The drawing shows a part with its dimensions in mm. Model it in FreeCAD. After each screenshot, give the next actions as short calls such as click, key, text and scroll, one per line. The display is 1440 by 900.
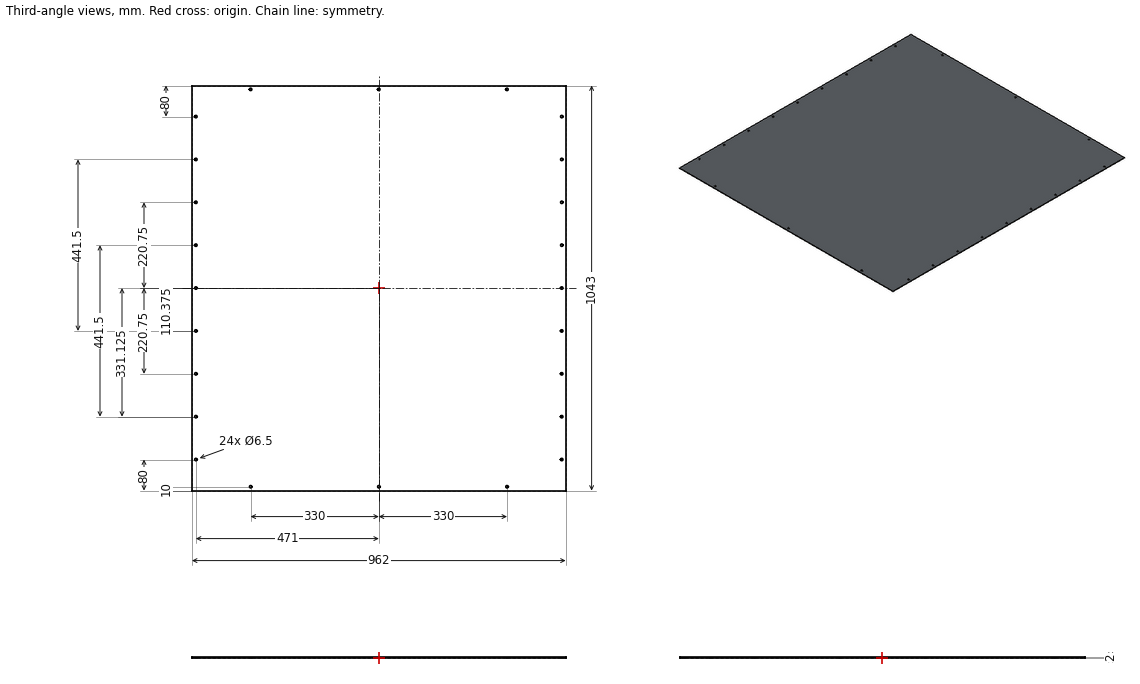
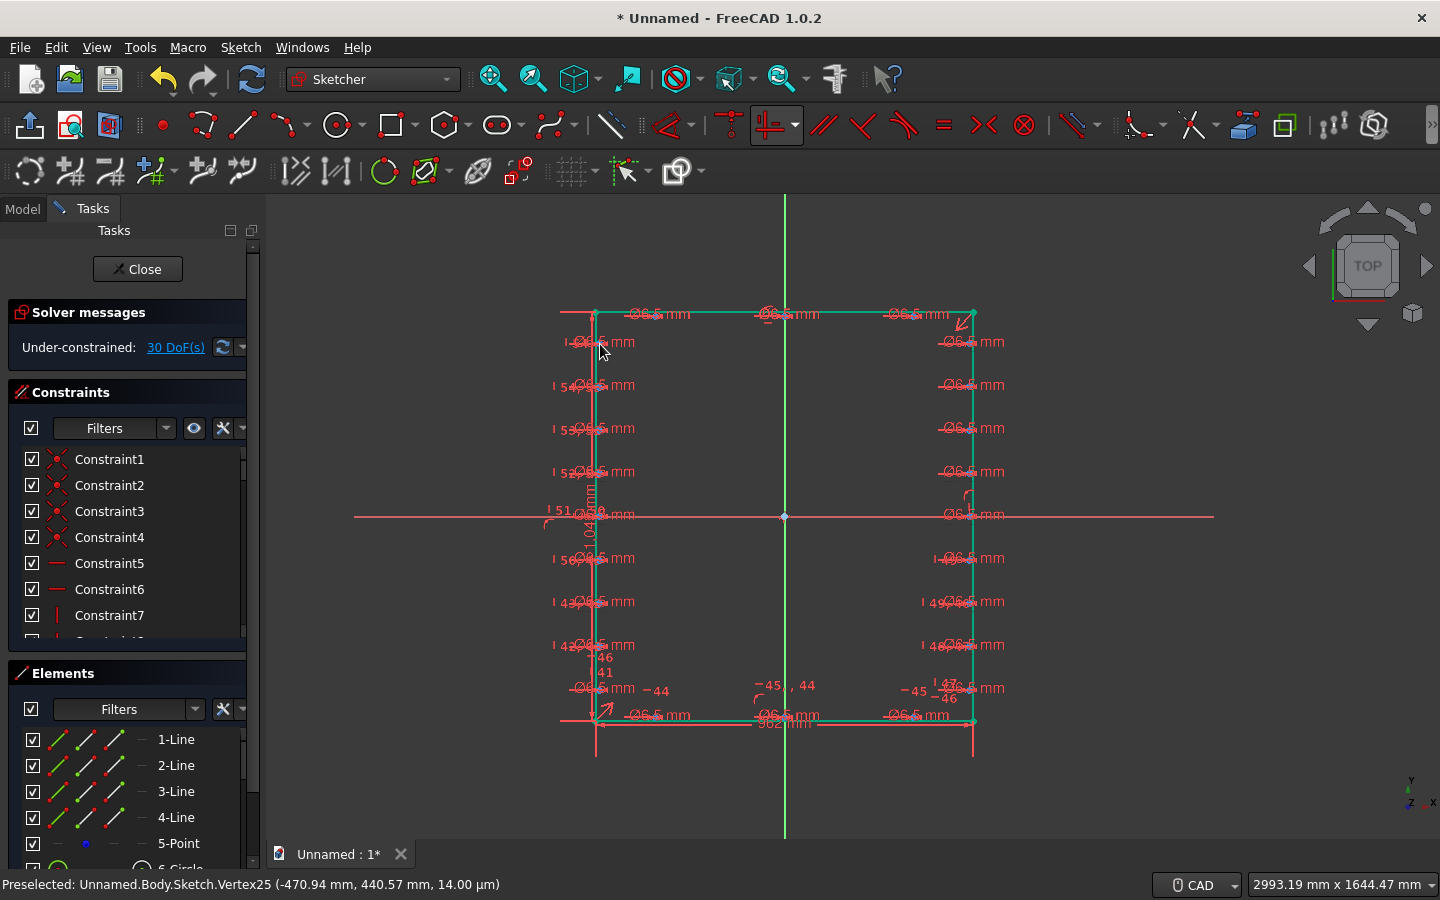
click(969, 560)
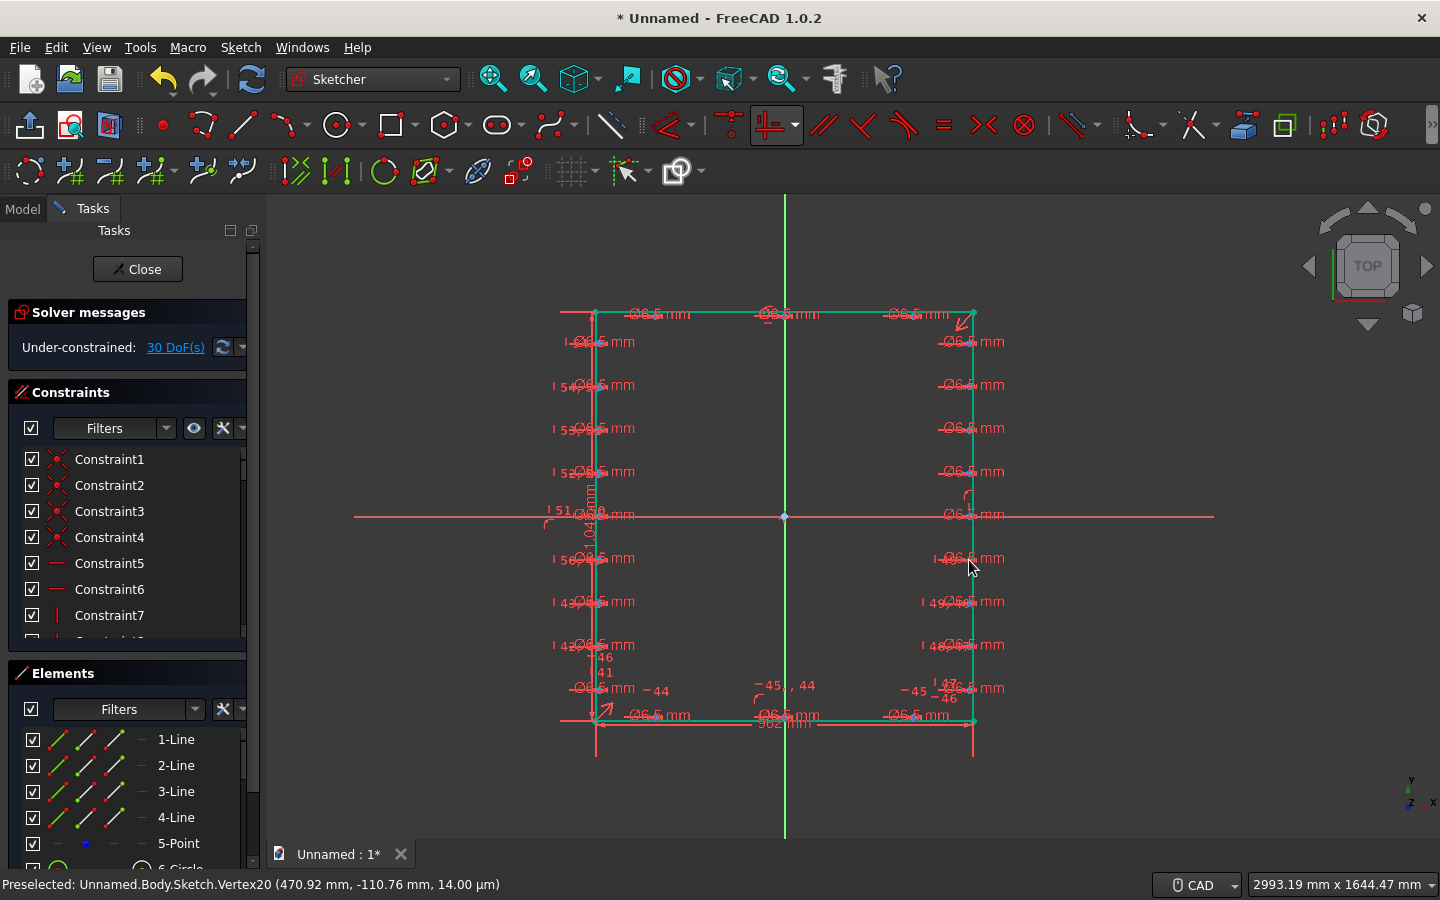
click(969, 517)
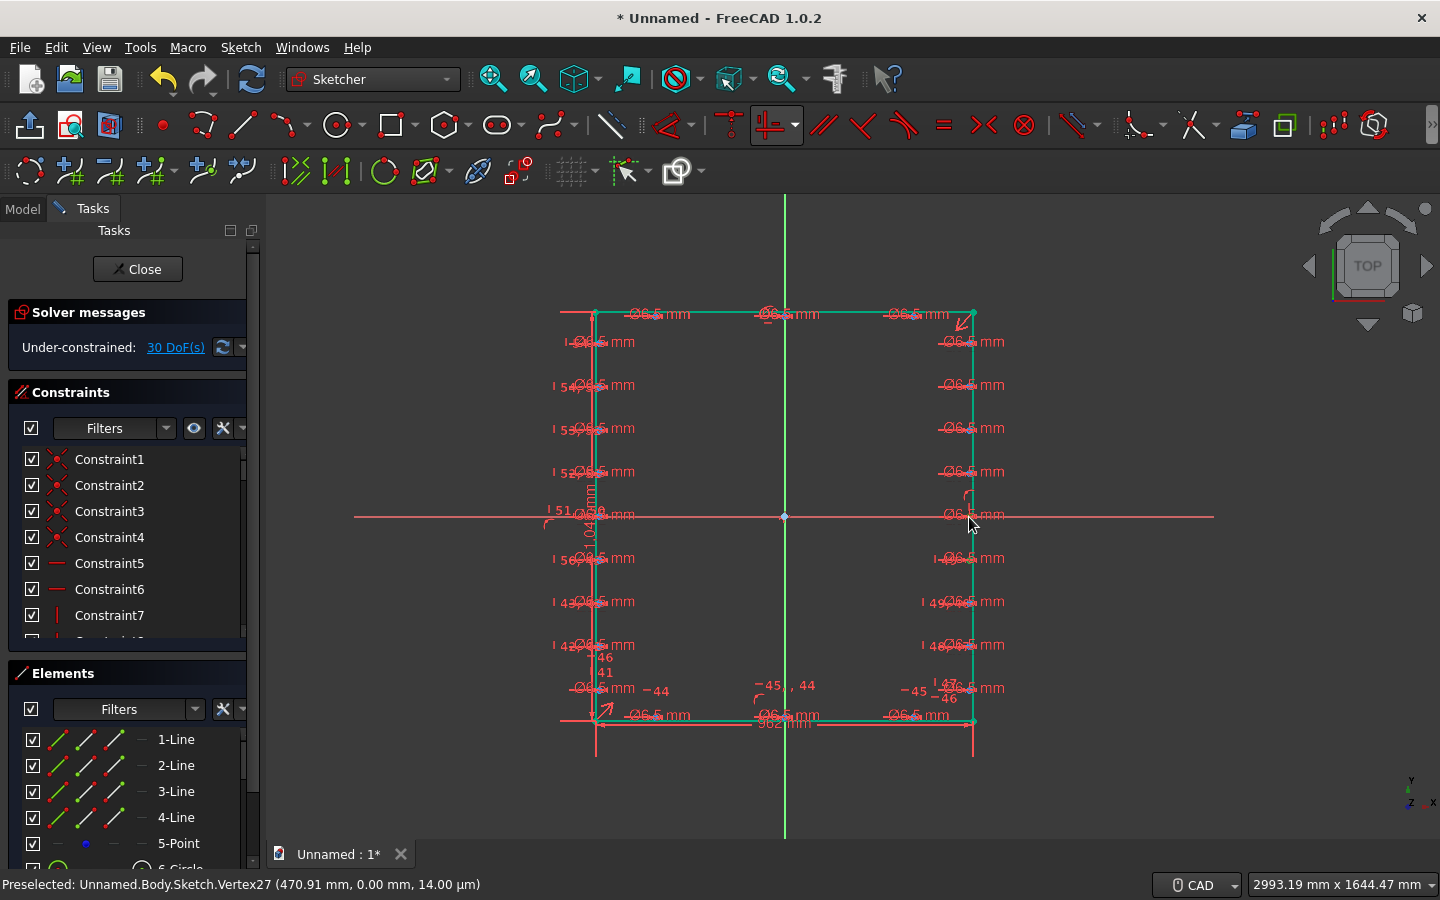
click(798, 126)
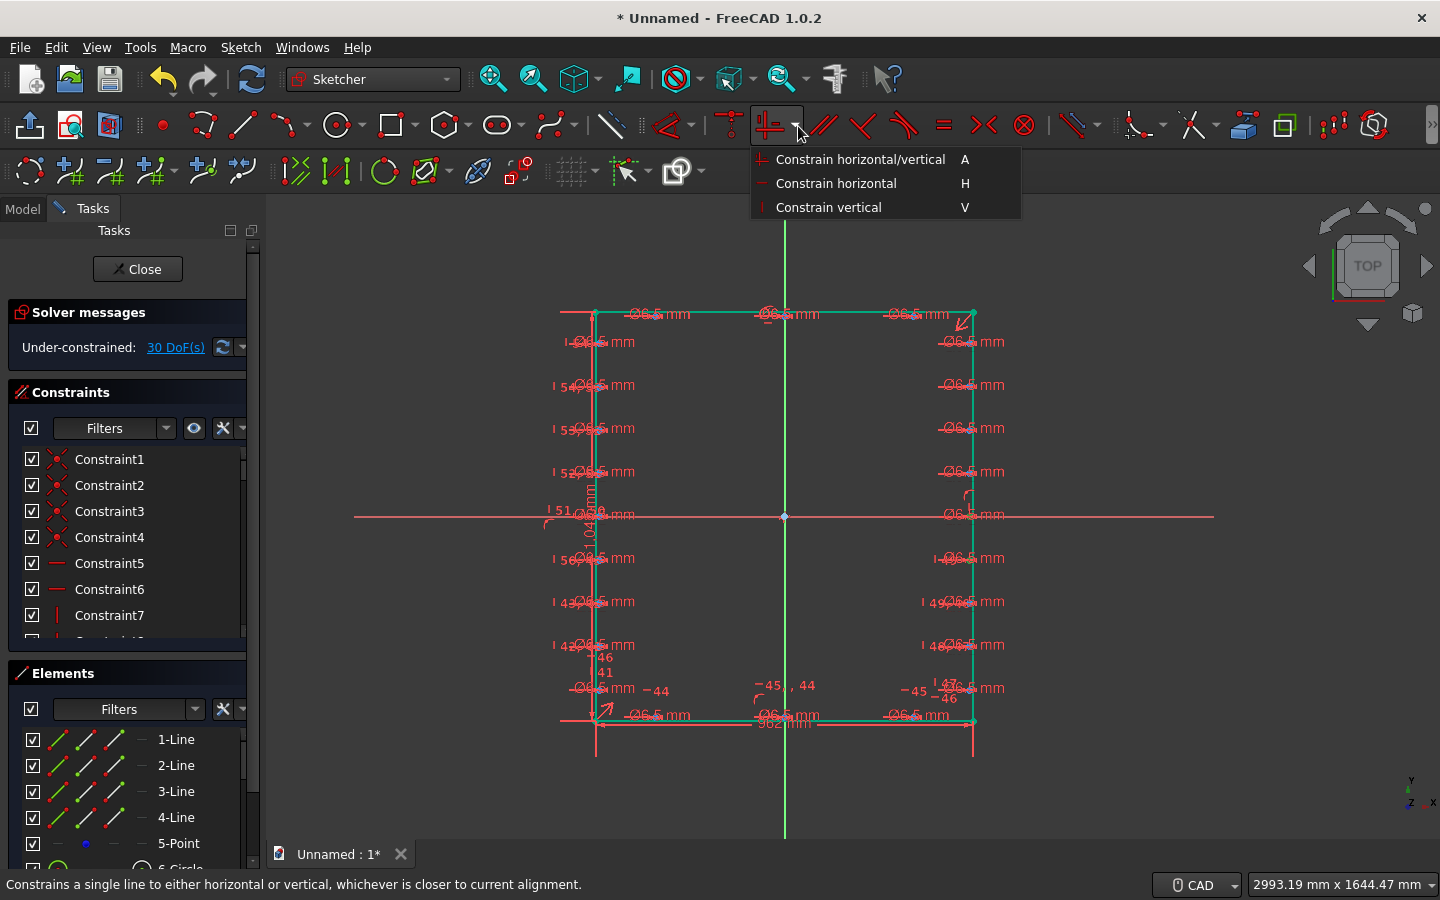
click(886, 207)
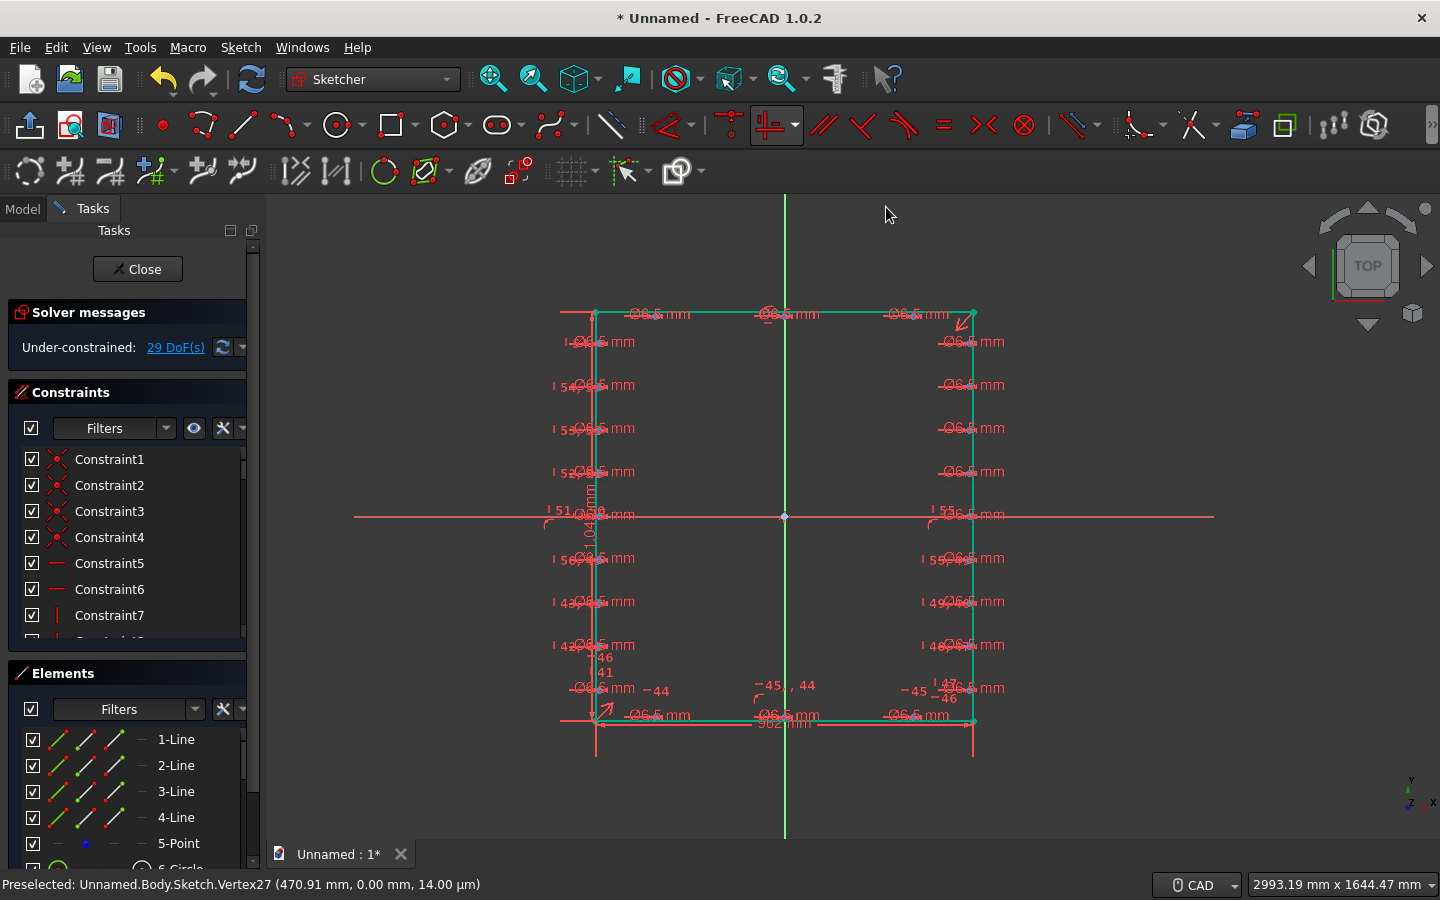
click(969, 517)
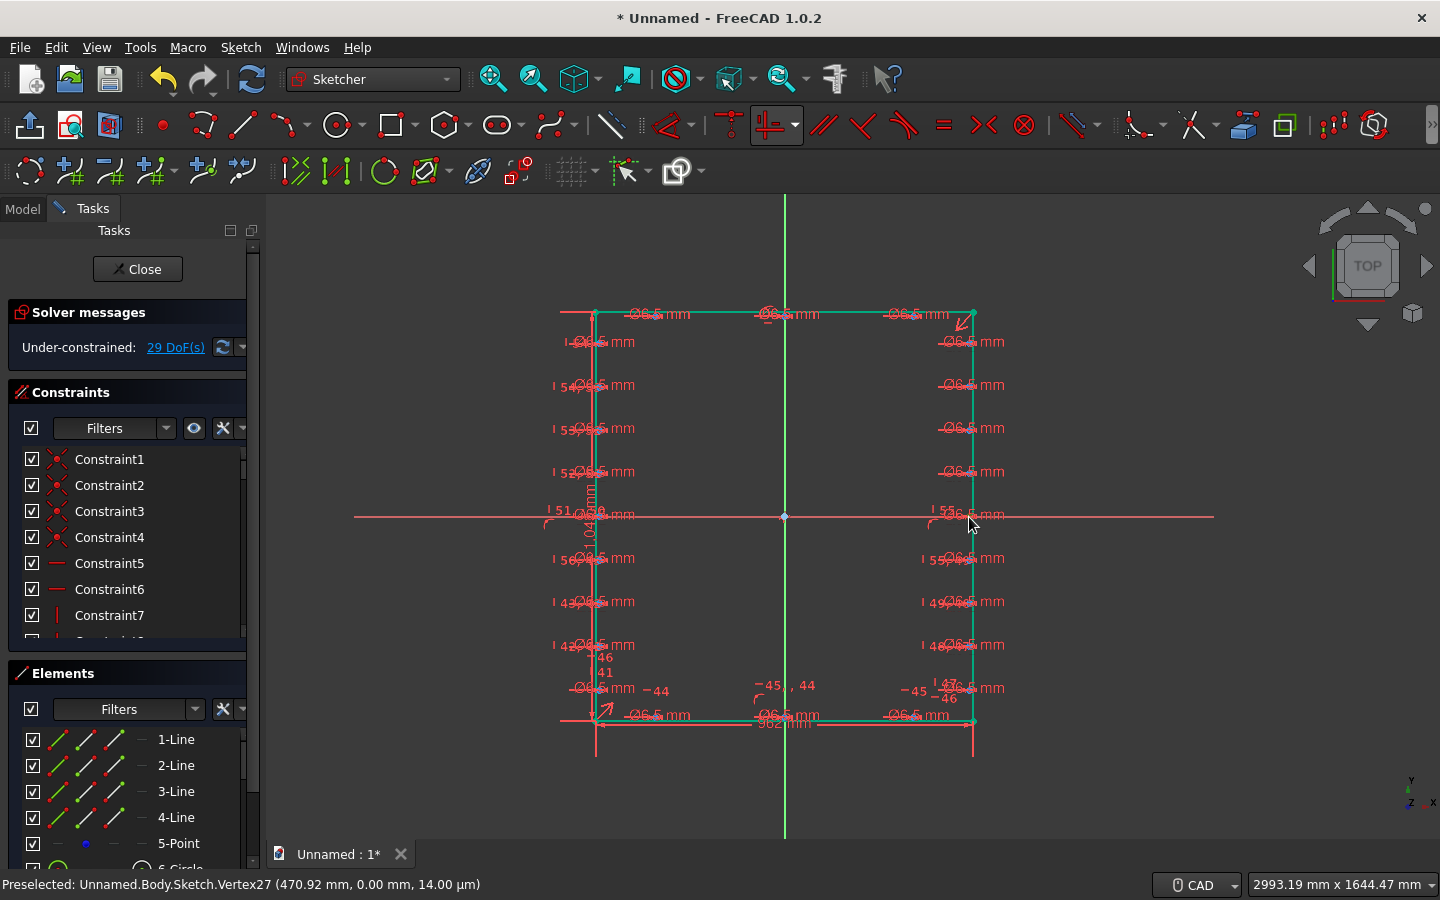
click(969, 474)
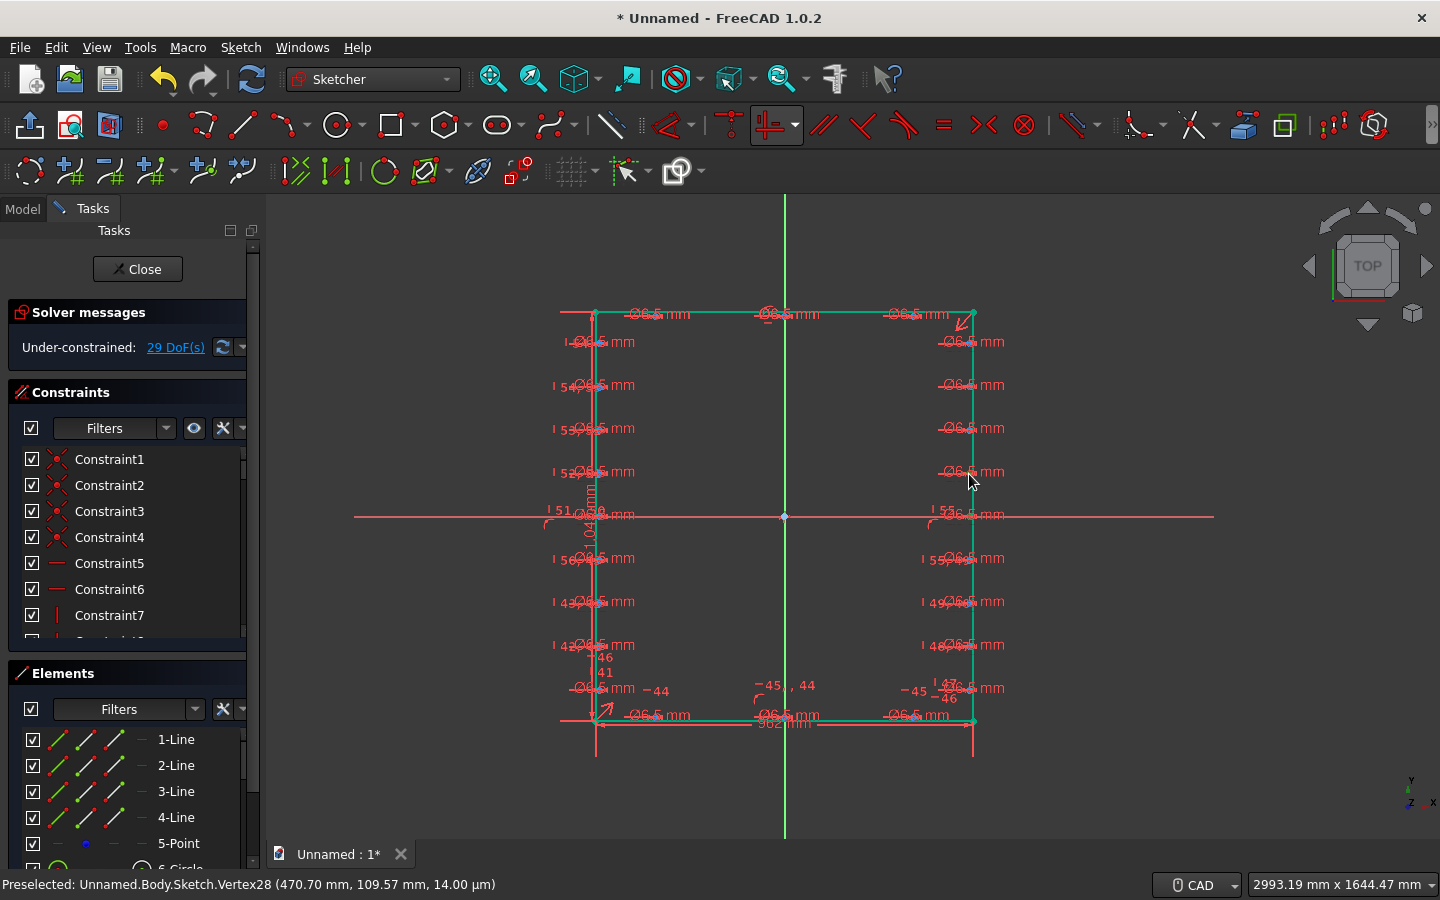
key(v)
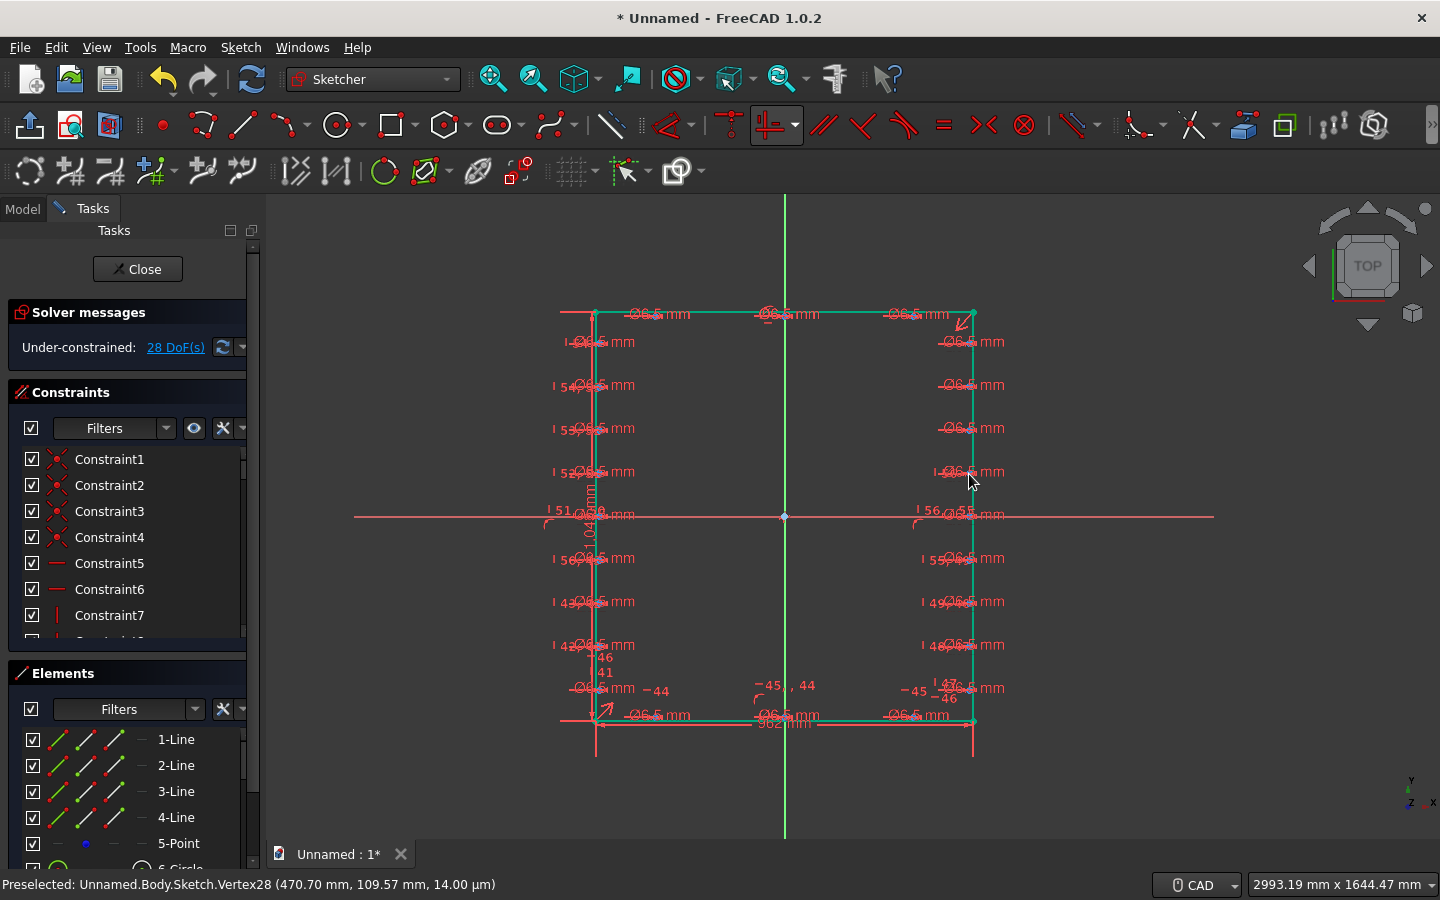
click(969, 474)